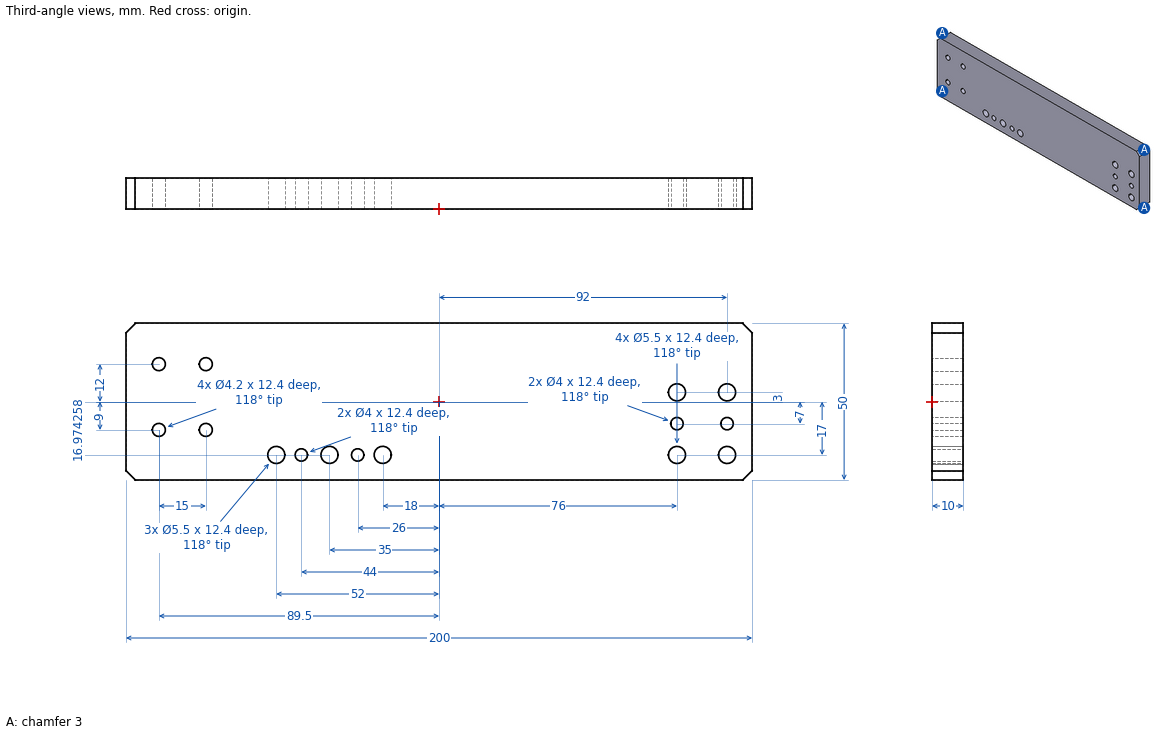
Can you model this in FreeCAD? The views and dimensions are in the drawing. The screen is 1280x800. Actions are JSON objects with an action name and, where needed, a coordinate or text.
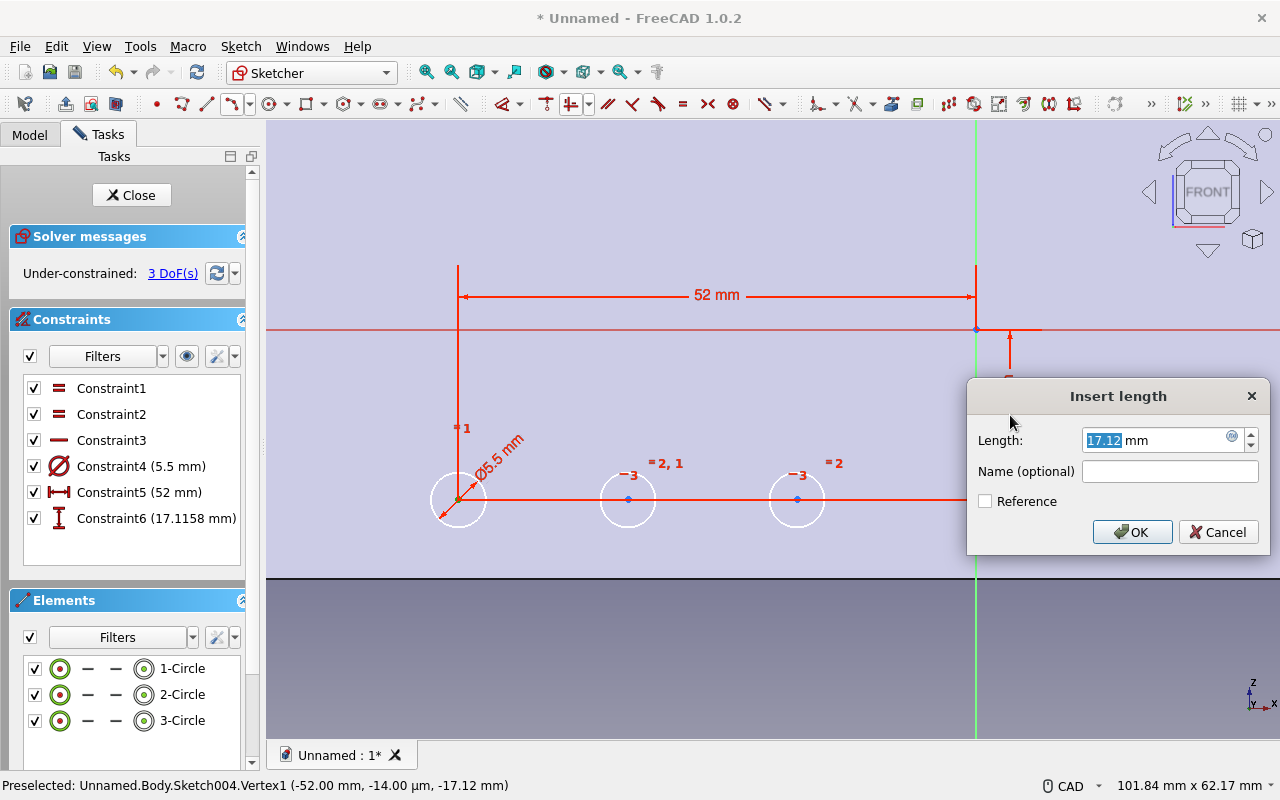
{"action": "type", "text": "17"}
{"action": "key", "text": "Return"}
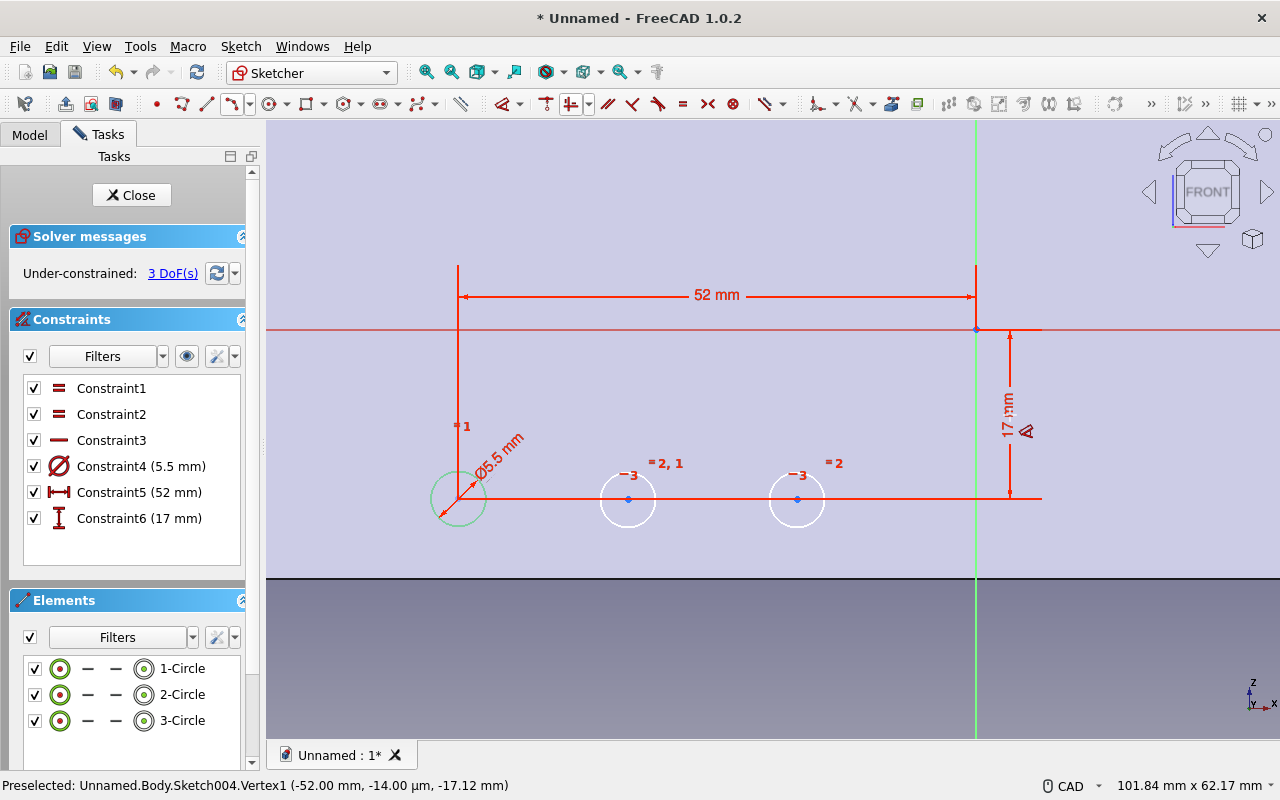
{"action": "left_click", "coordinate": [628, 500]}
{"action": "left_click", "coordinate": [802, 296]}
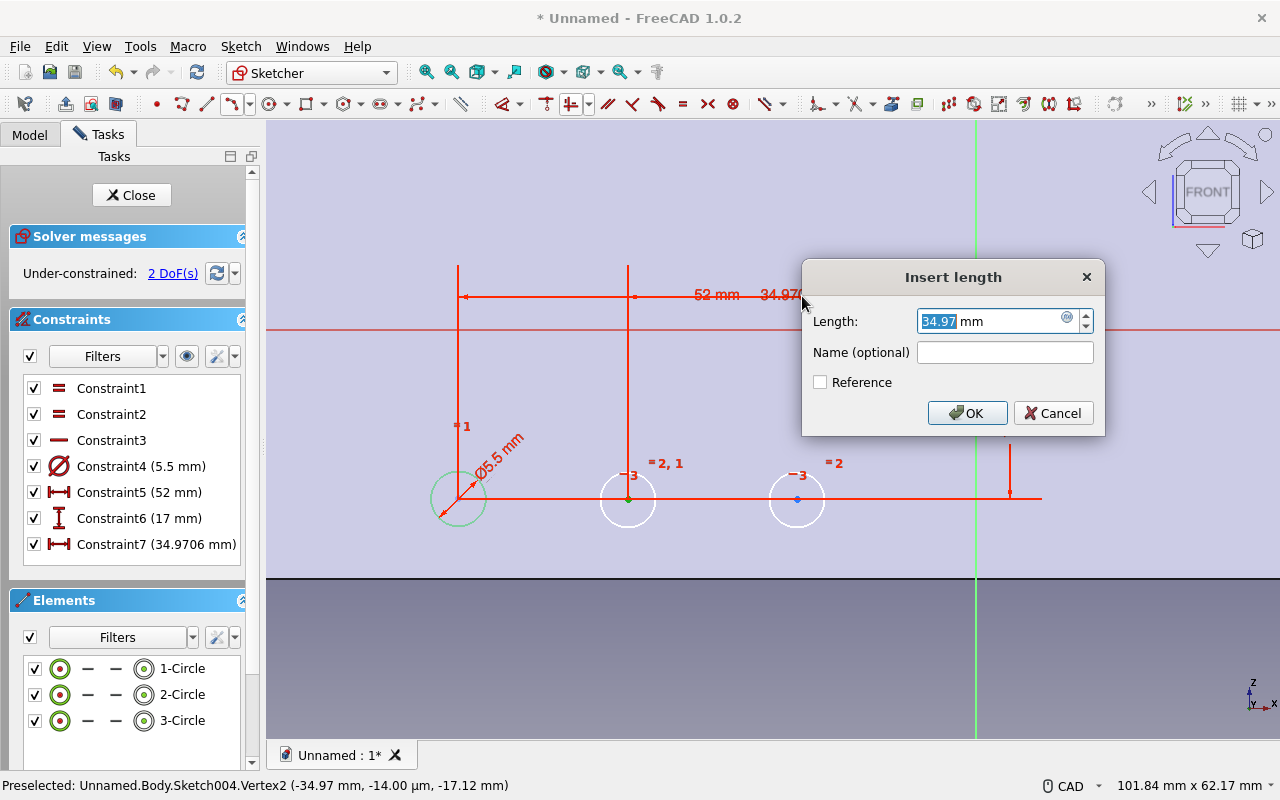
{"action": "type", "text": "35"}
{"action": "key", "text": "Return"}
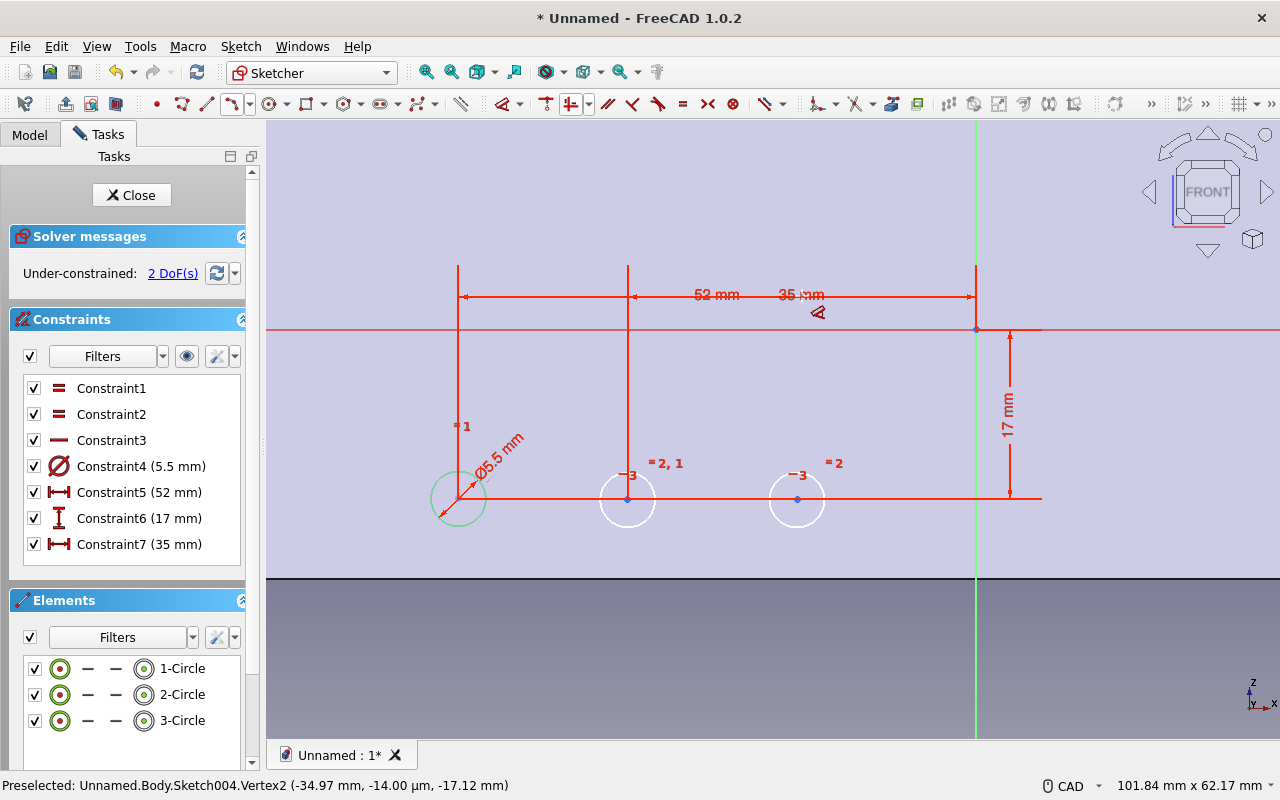
{"action": "left_click", "coordinate": [797, 500]}
{"action": "left_click", "coordinate": [887, 296]}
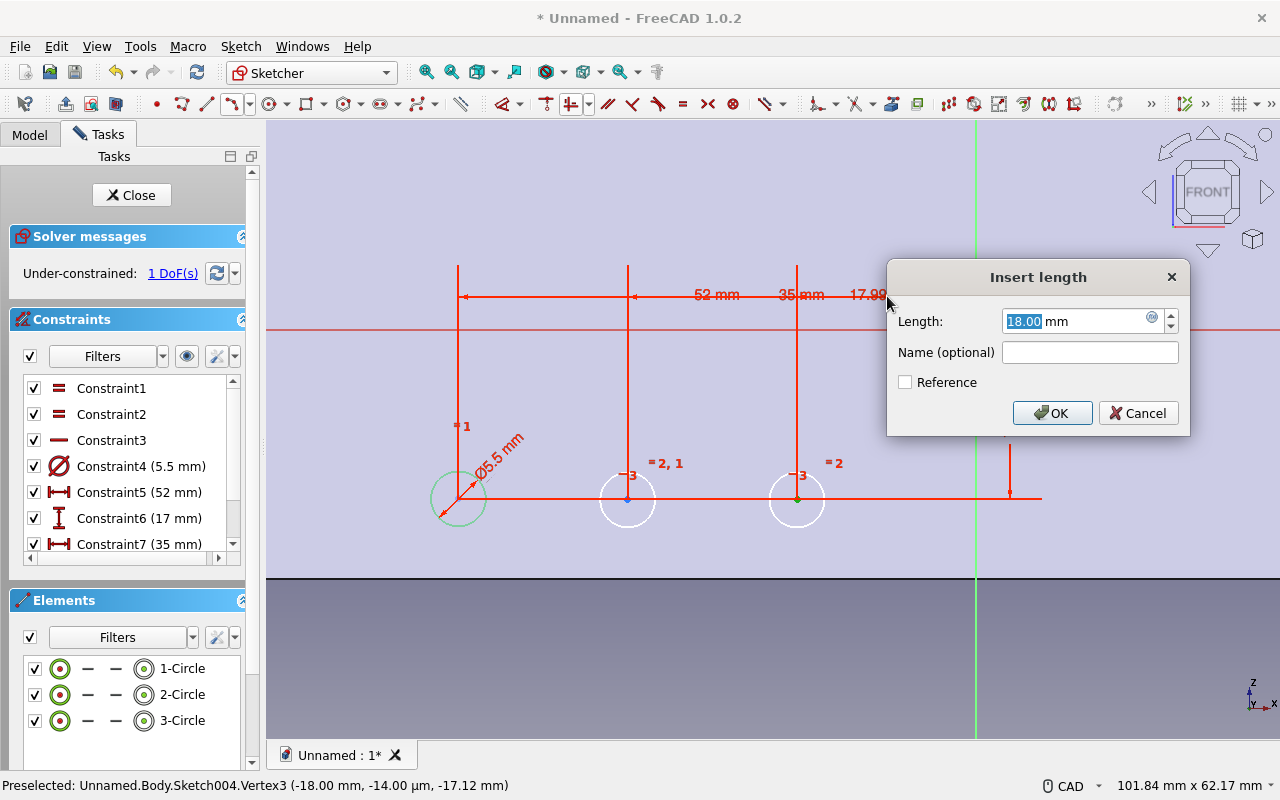
{"action": "type", "text": "18"}
{"action": "key", "text": "Return"}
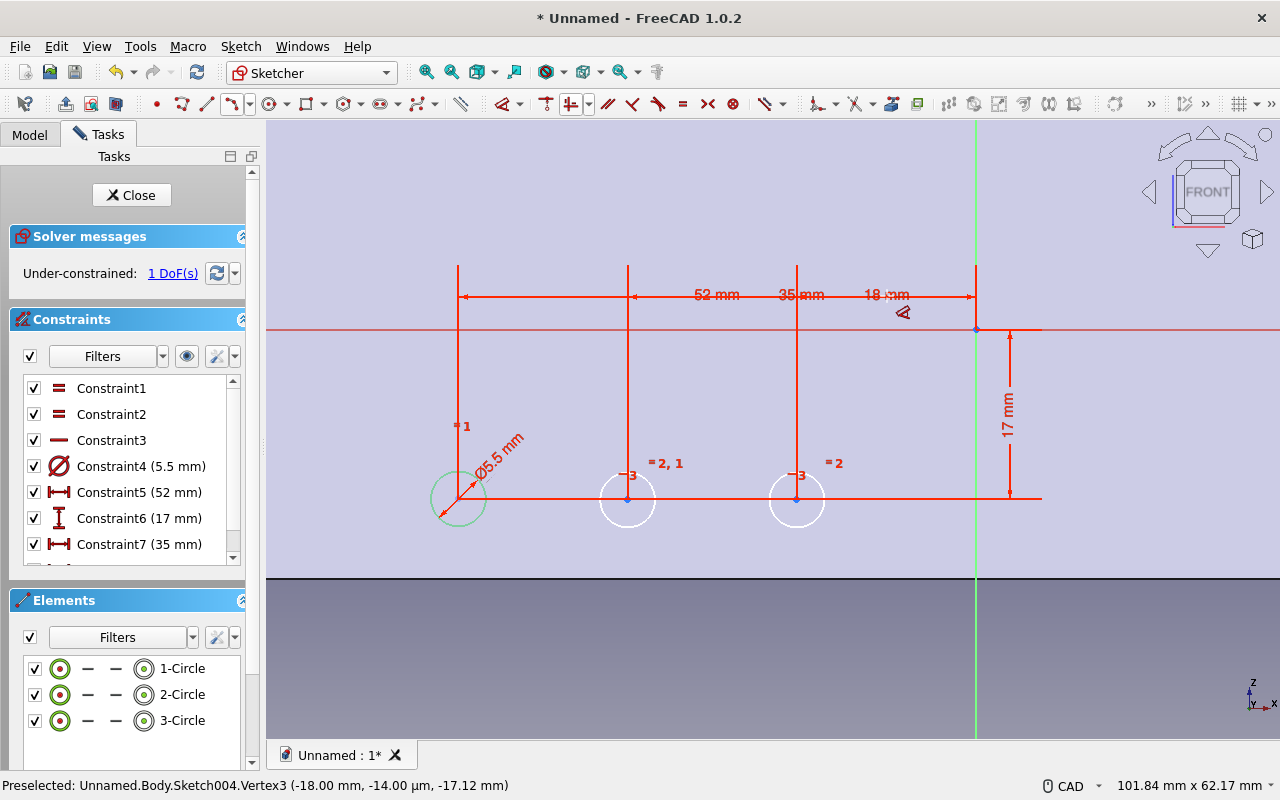
{"action": "left_click", "coordinate": [628, 500]}
{"action": "left_click", "coordinate": [1010, 376]}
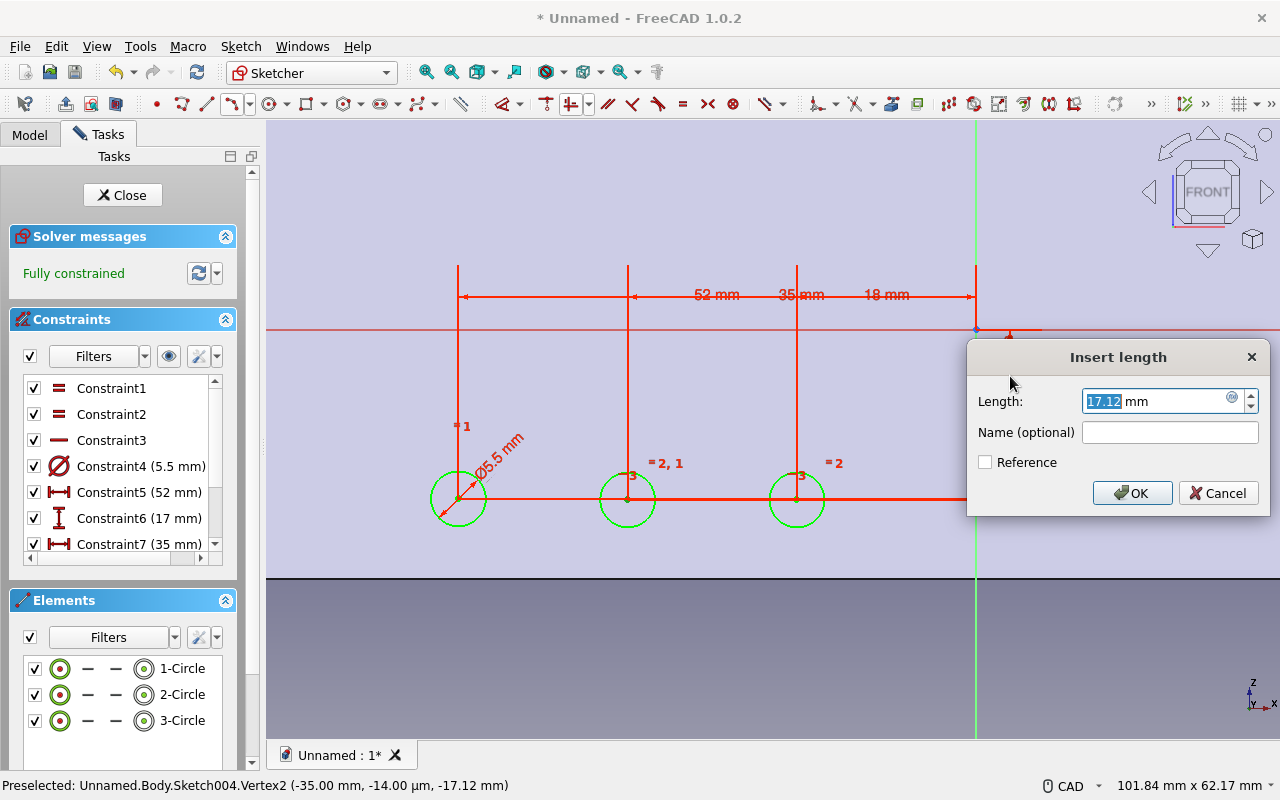
{"action": "type", "text": "16.974258"}
{"action": "key", "text": "Return"}
{"action": "key", "text": "Escape"}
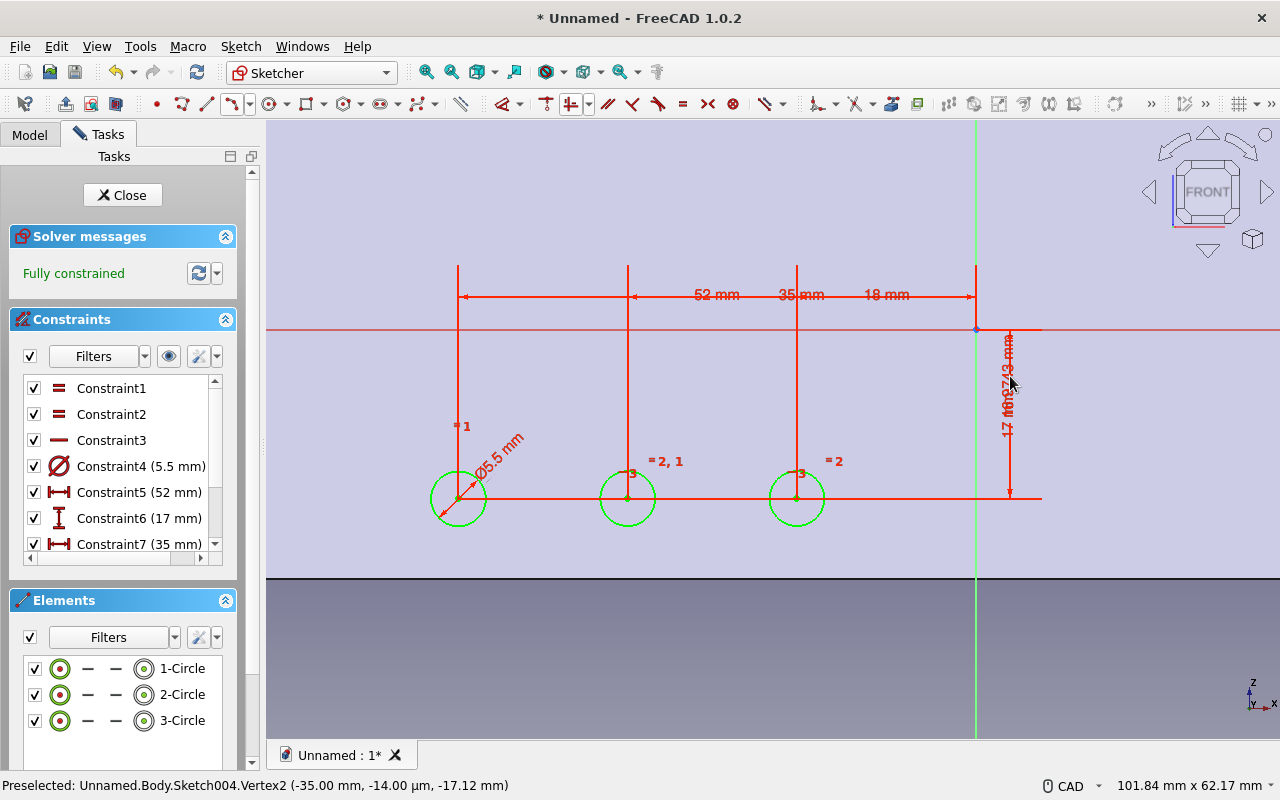
{"action": "left_click", "coordinate": [123, 195]}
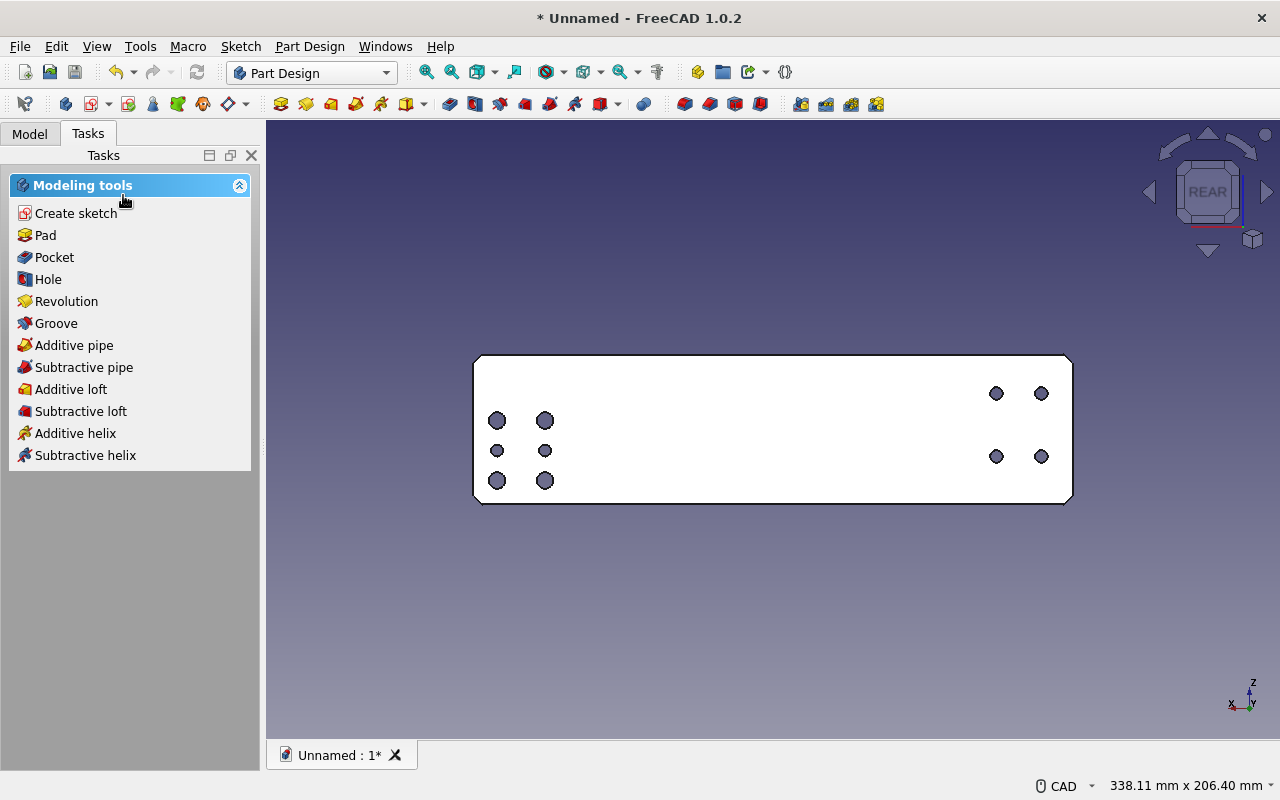
{"action": "left_click", "coordinate": [475, 104]}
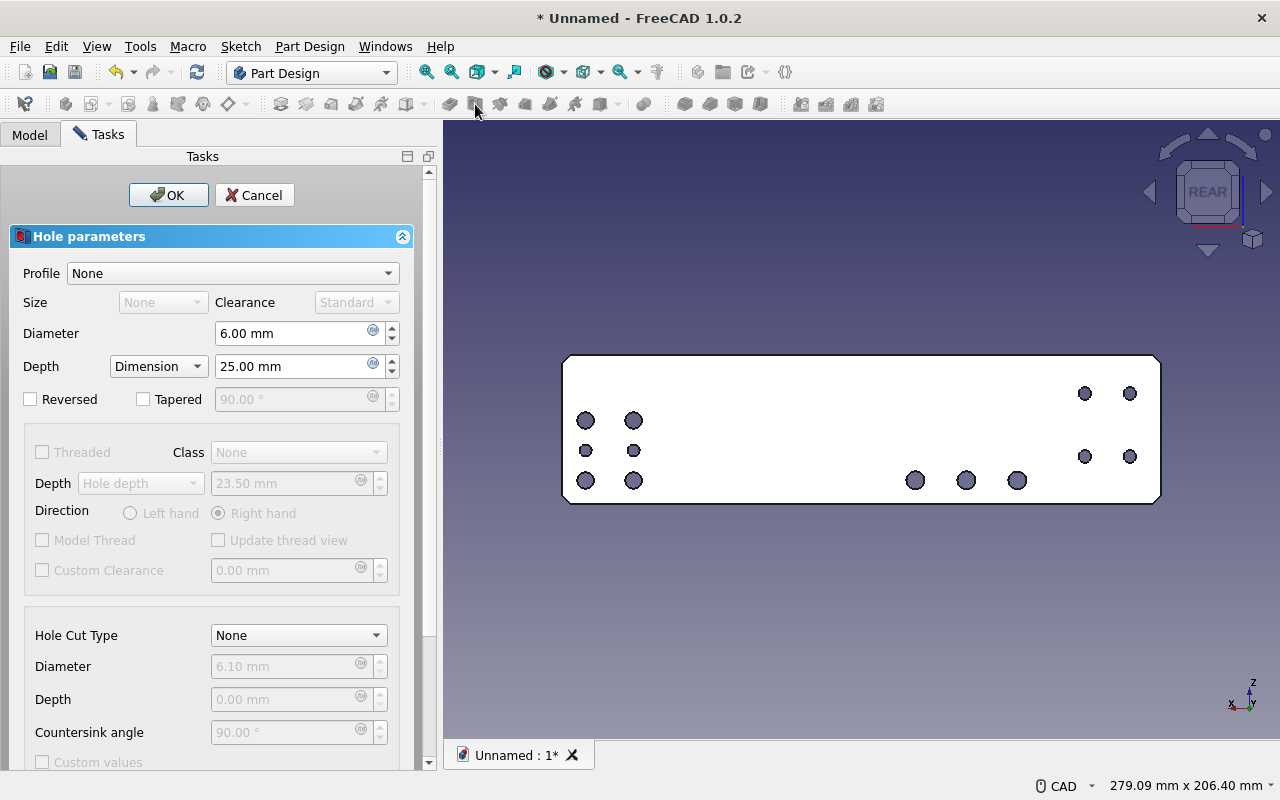
{"action": "triple_click", "coordinate": [300, 334]}